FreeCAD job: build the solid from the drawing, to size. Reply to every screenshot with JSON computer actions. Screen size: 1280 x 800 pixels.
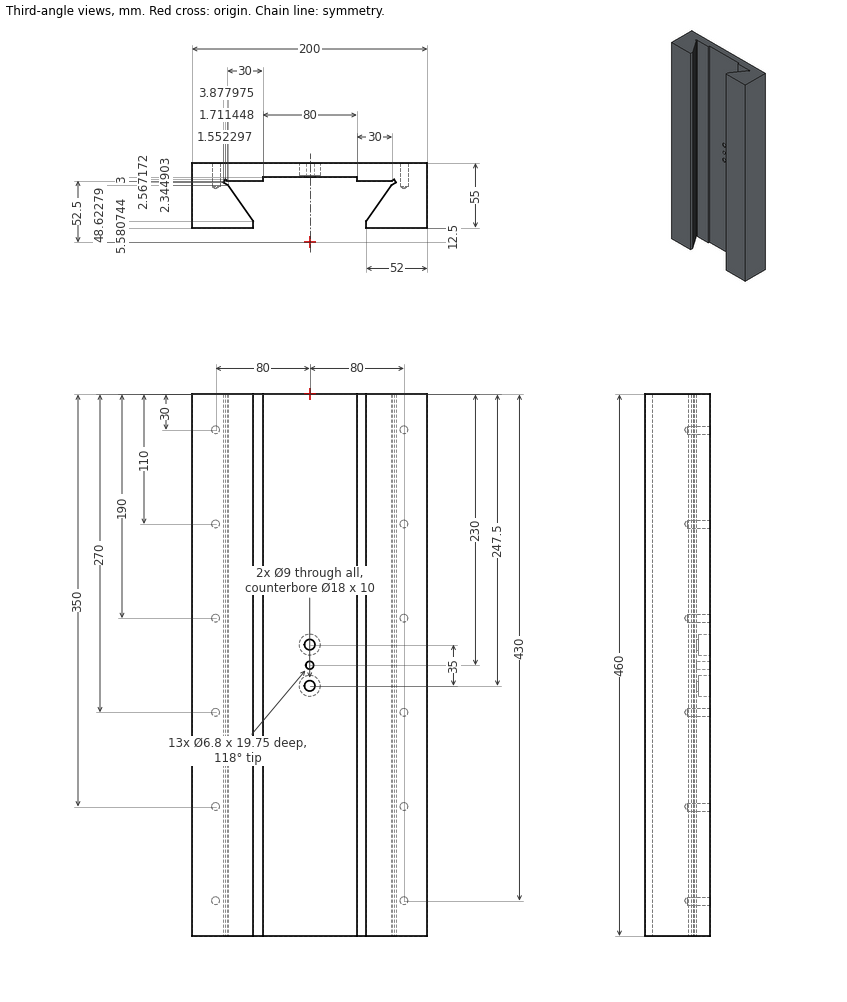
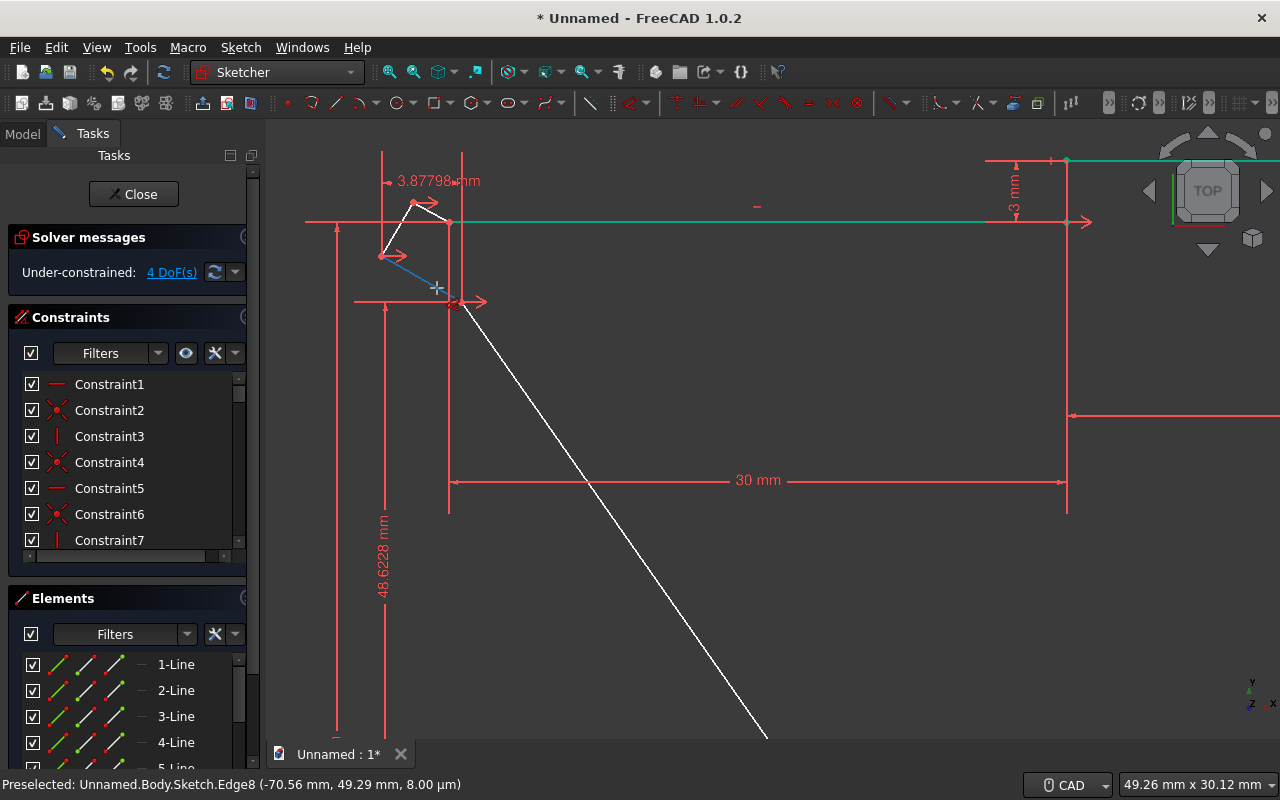
{"action": "left_click", "coordinate": [438, 288]}
{"action": "left_click", "coordinate": [348, 279]}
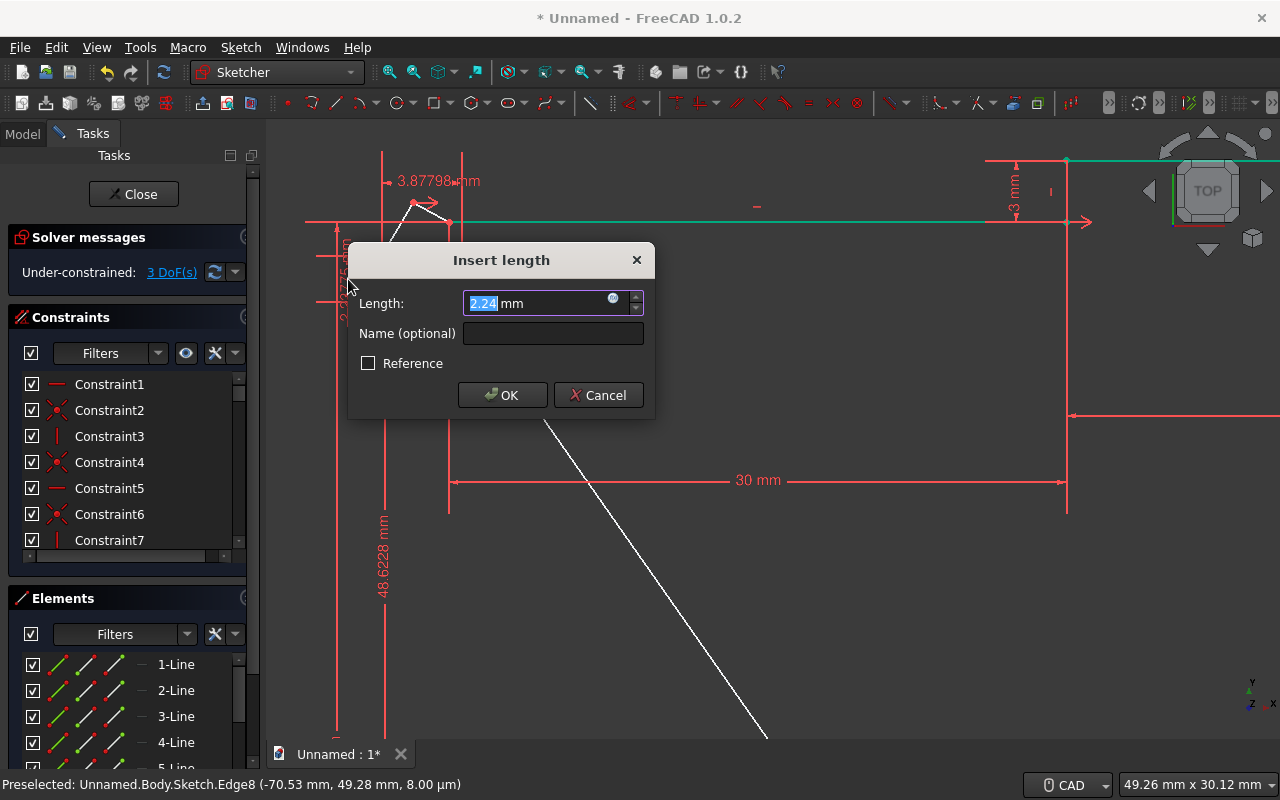
{"action": "type", "text": "2.344903"}
{"action": "key", "text": "Return"}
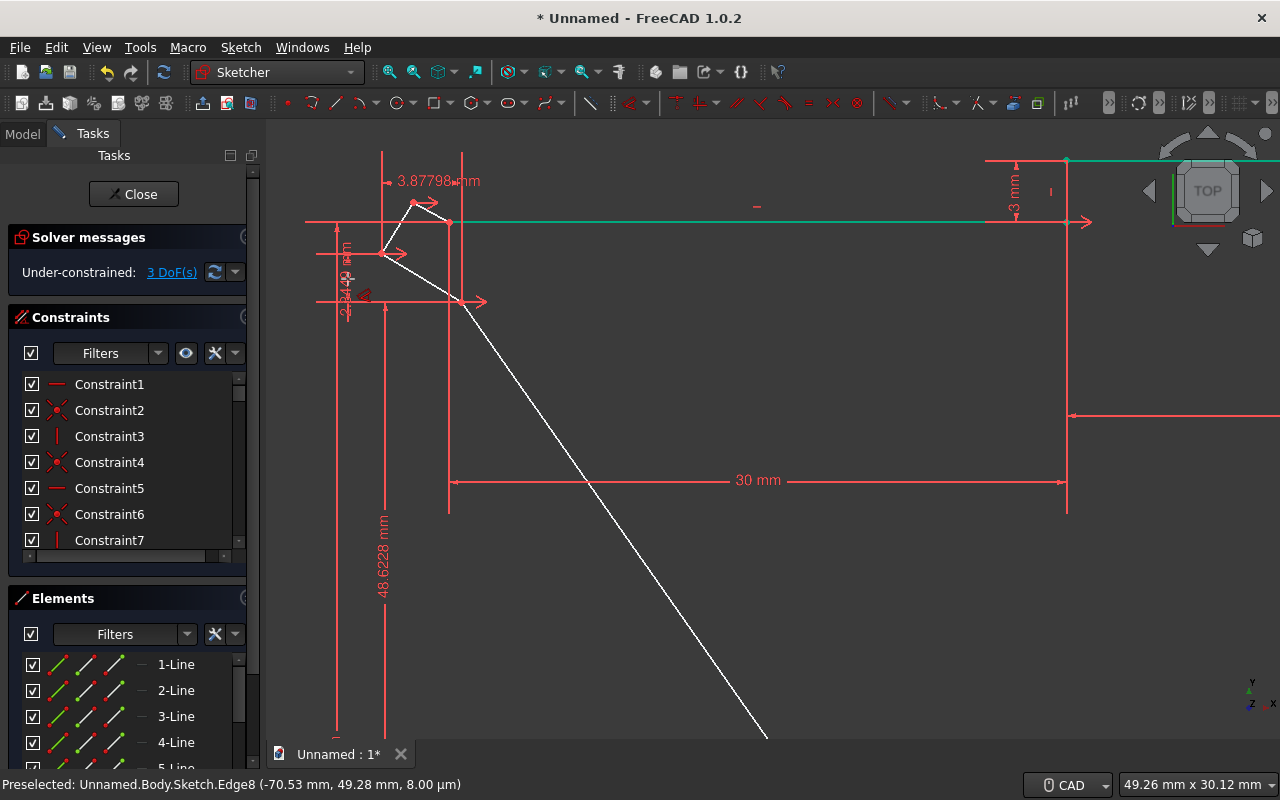
{"action": "scroll", "coordinate": [391, 239], "scroll_direction": "up", "scroll_amount": 2}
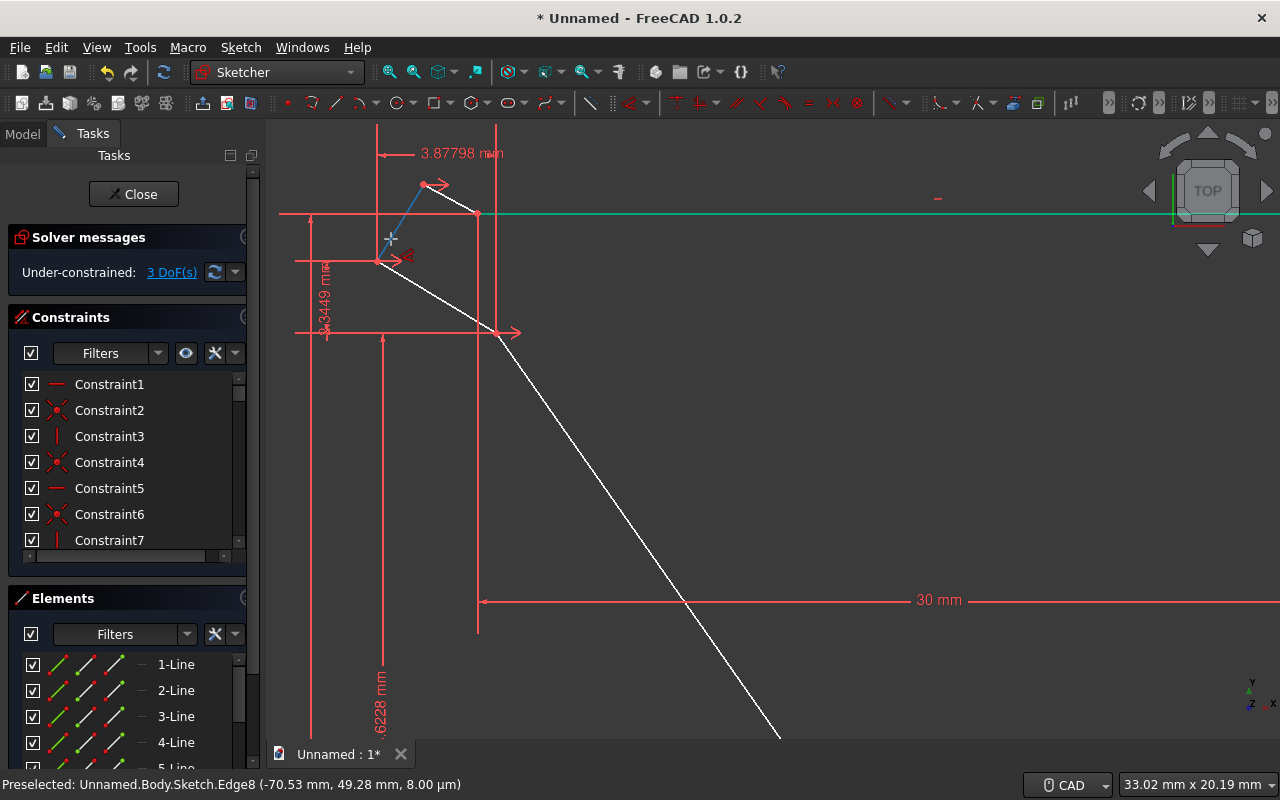
{"action": "left_click", "coordinate": [391, 238]}
{"action": "left_click", "coordinate": [390, 151]}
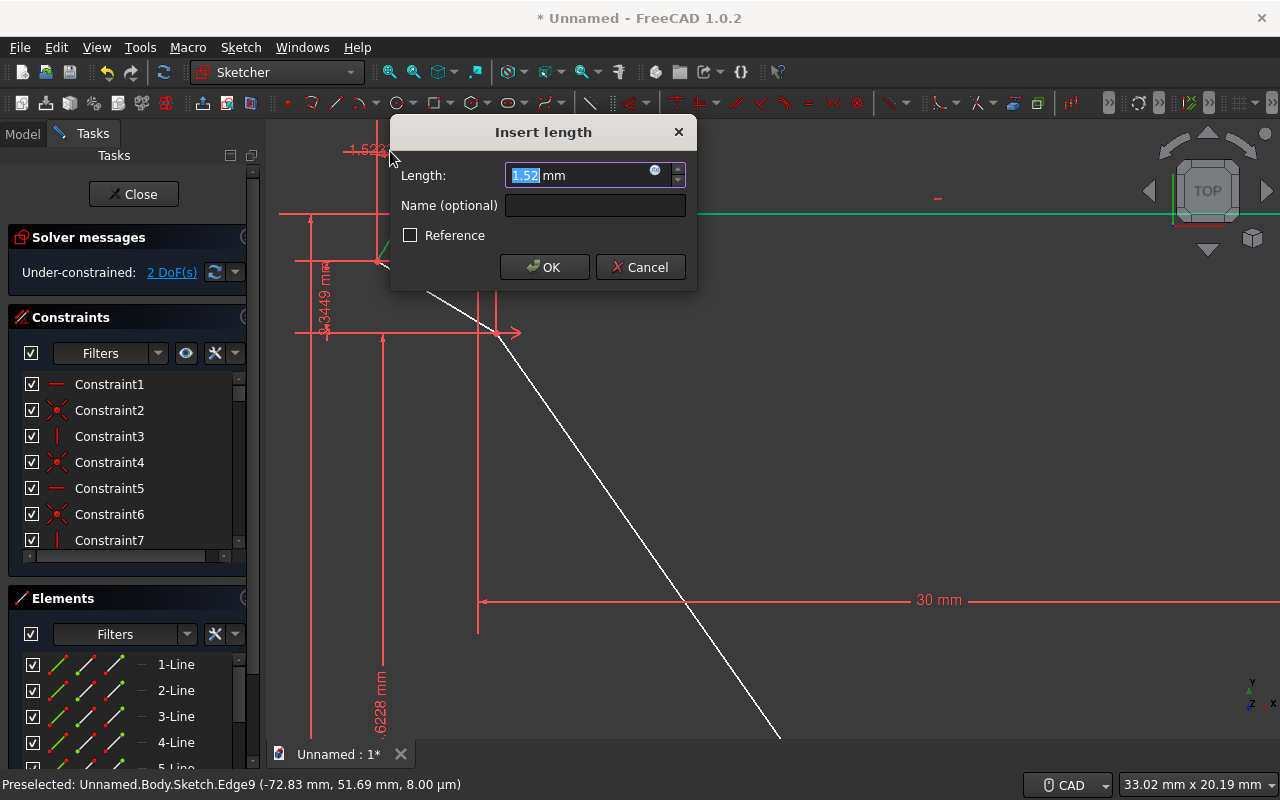
{"action": "type", "text": "1.552297"}
{"action": "key", "text": "Return"}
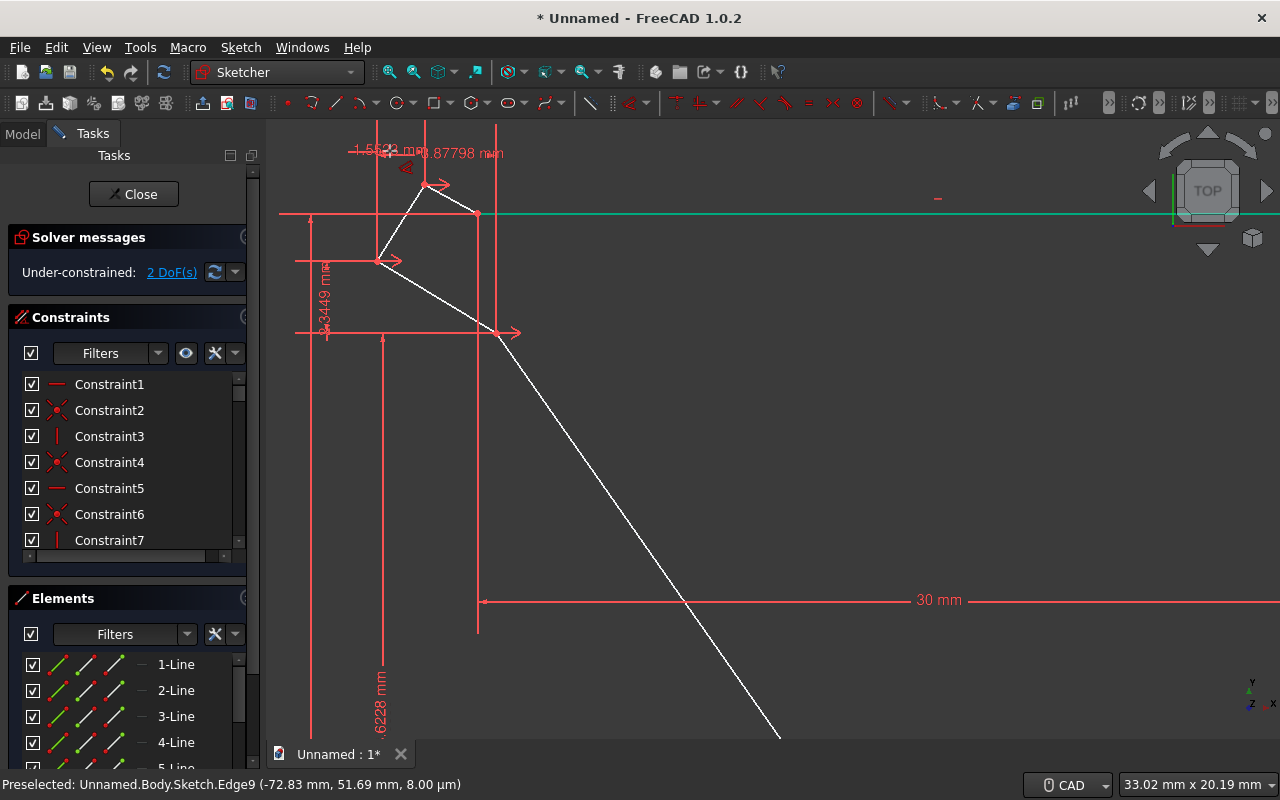
{"action": "left_click", "coordinate": [391, 238]}
{"action": "left_click", "coordinate": [343, 223]}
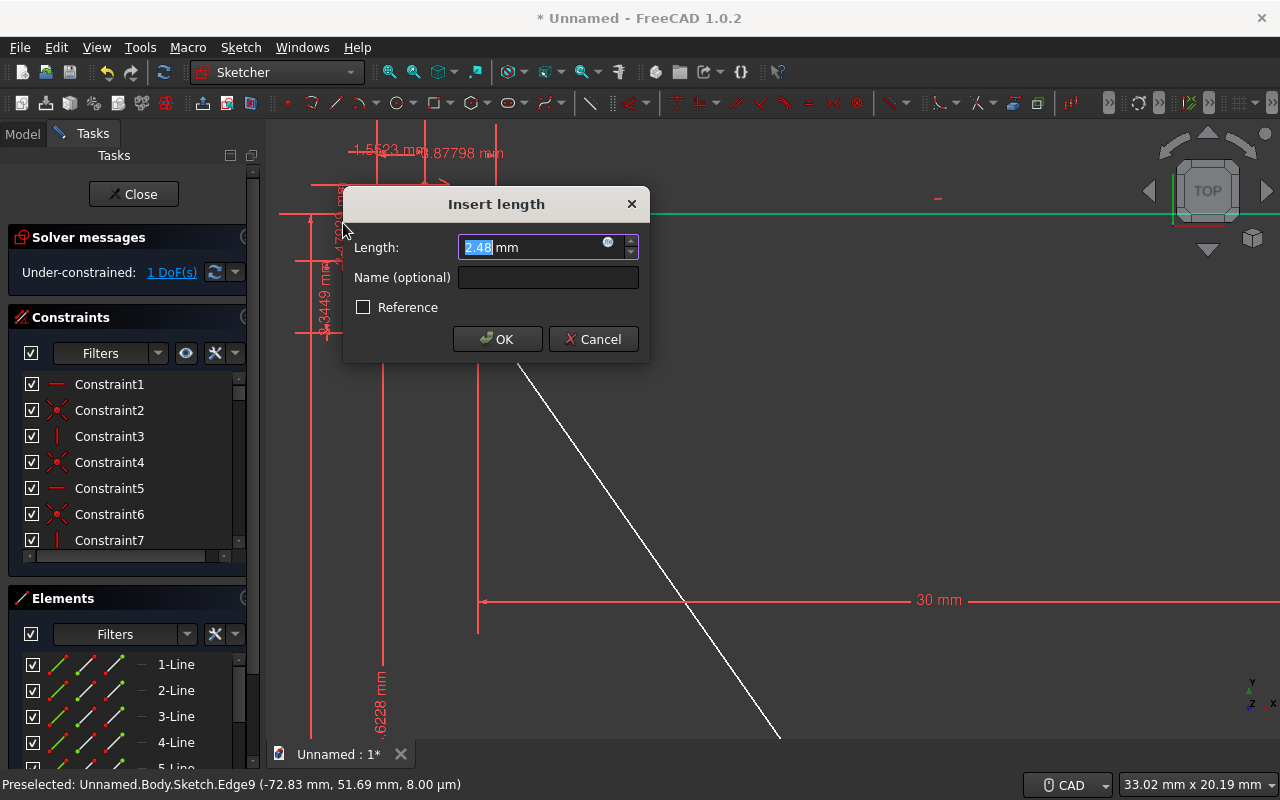
{"action": "type", "text": "2.567172"}
{"action": "key", "text": "Return"}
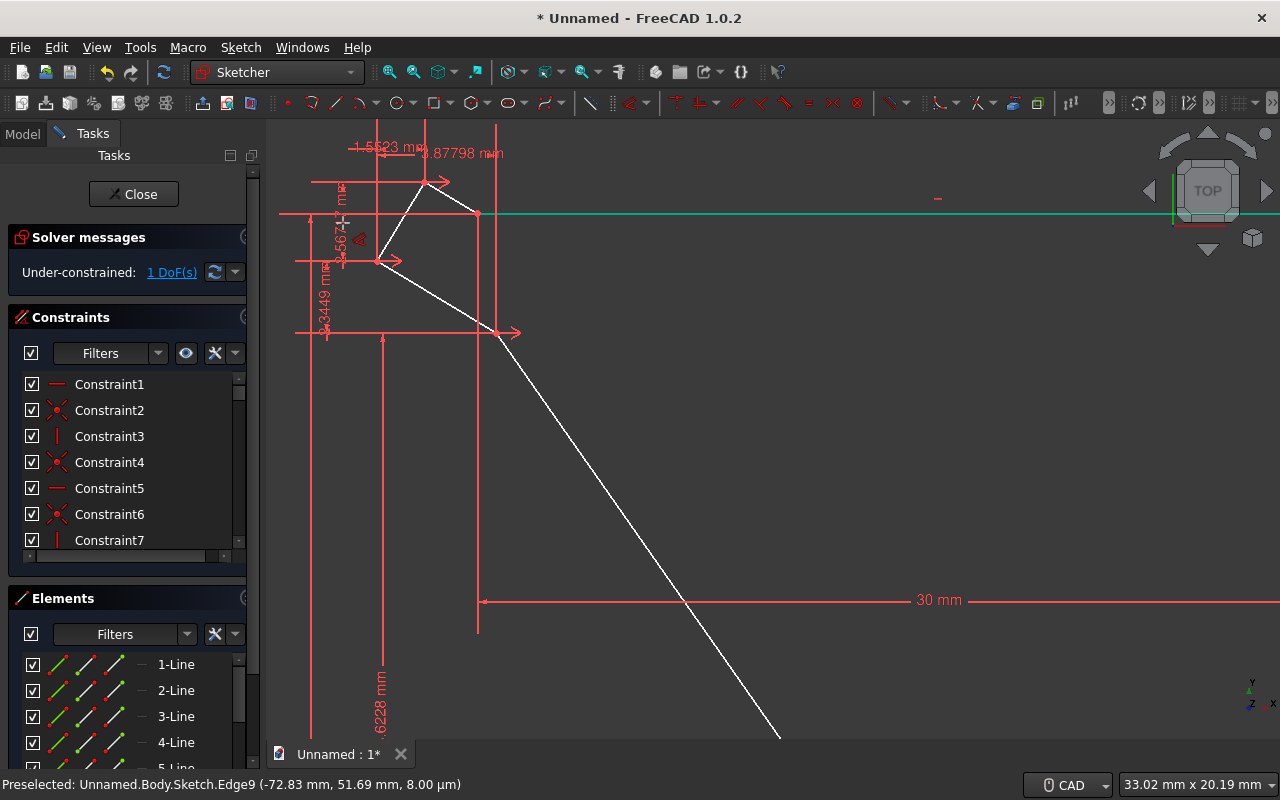
{"action": "left_click", "coordinate": [441, 192]}
{"action": "left_click", "coordinate": [451, 248]}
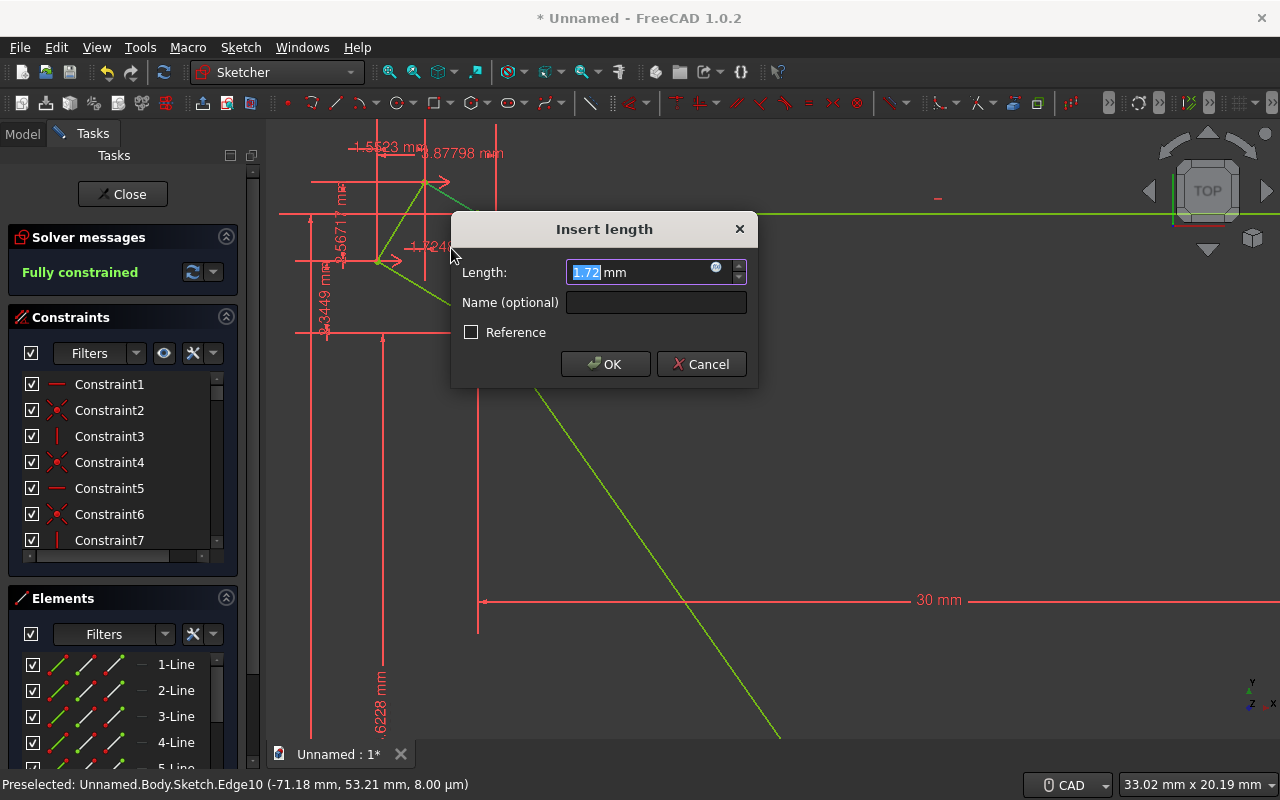
{"action": "type", "text": "1.711448"}
{"action": "key", "text": "Return"}
{"action": "key", "text": "Escape"}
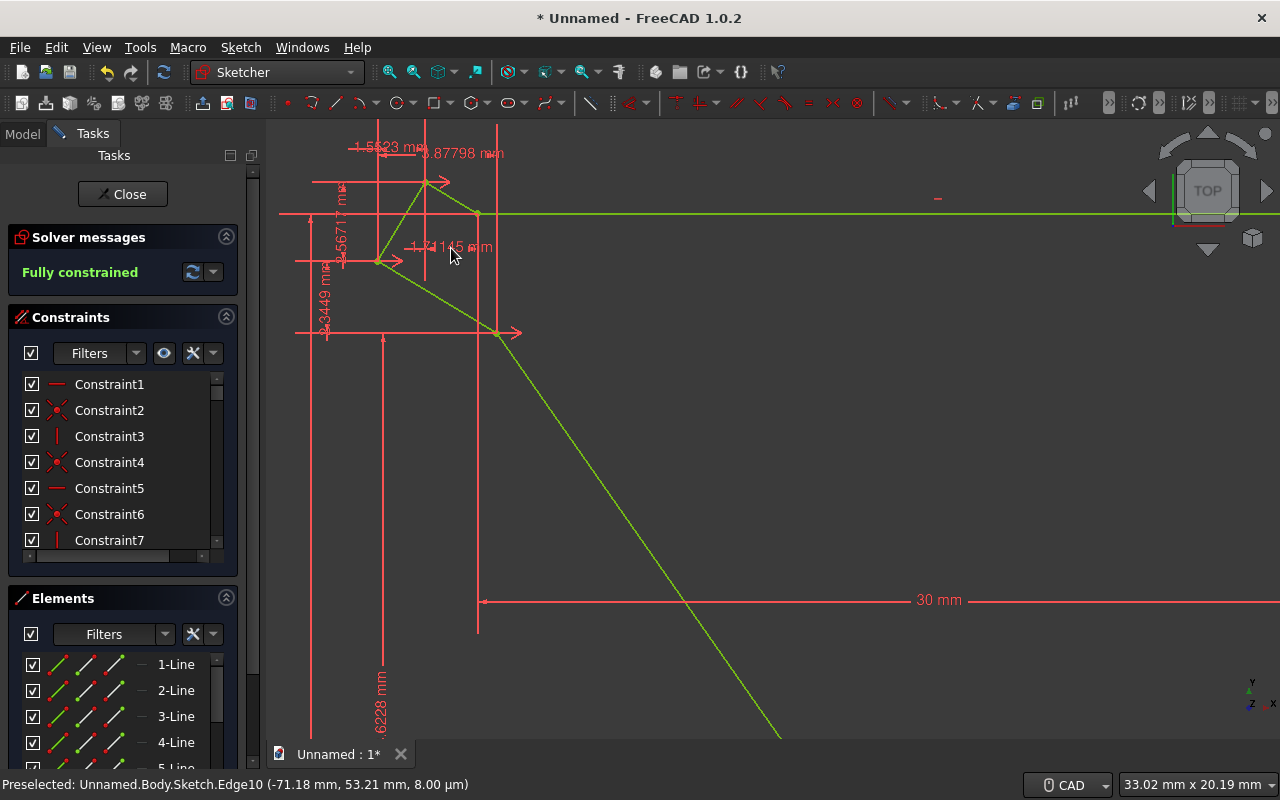
{"action": "left_click", "coordinate": [123, 194]}